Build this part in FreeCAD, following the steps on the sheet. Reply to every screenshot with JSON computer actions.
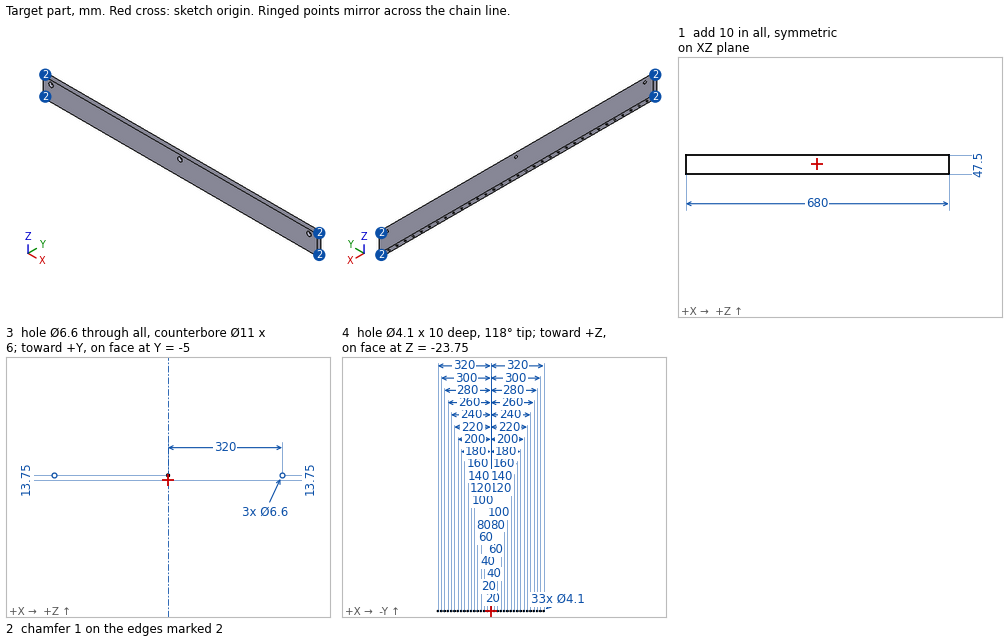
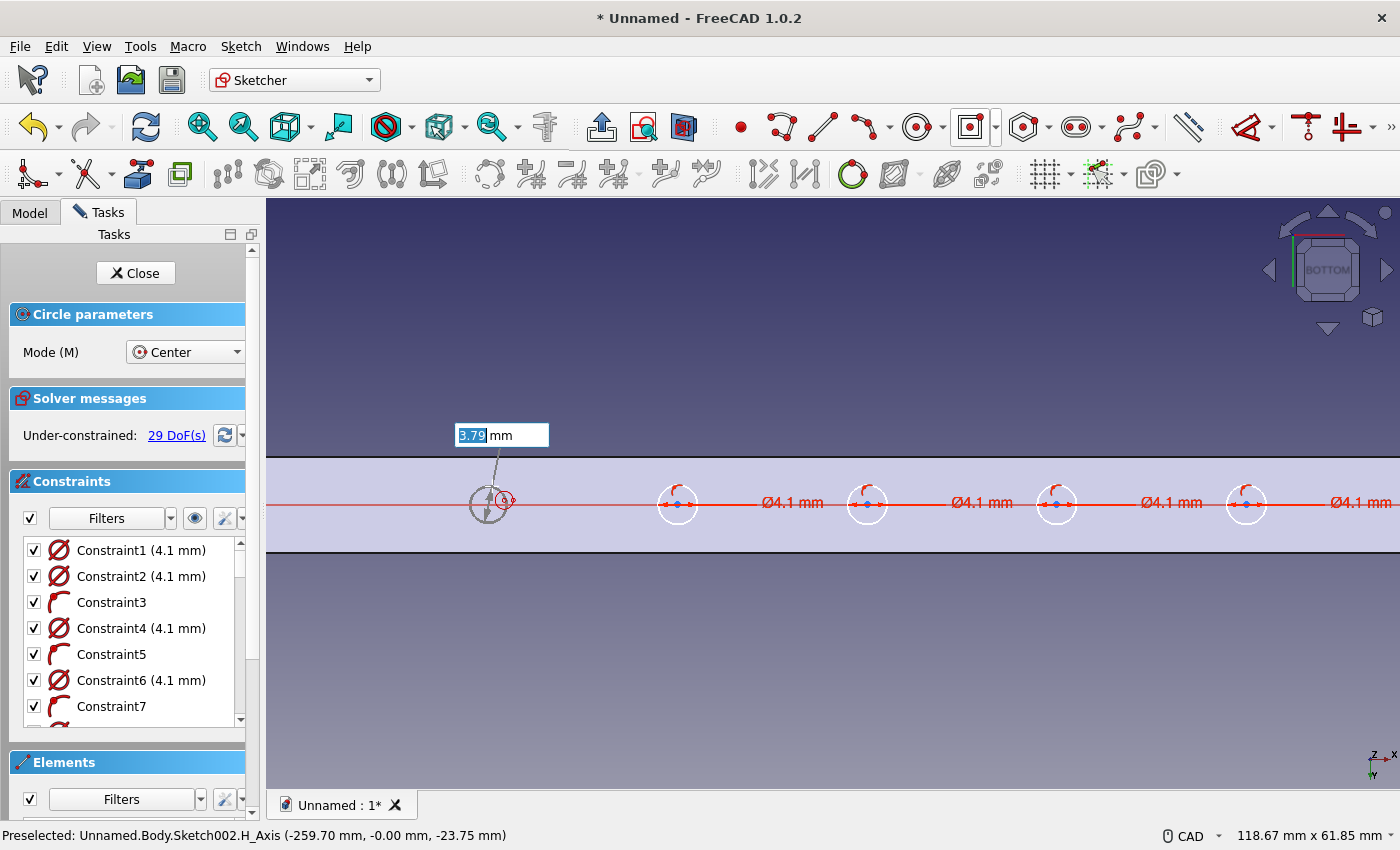
{"action": "type", "text": "4.1"}
{"action": "key", "text": "Return"}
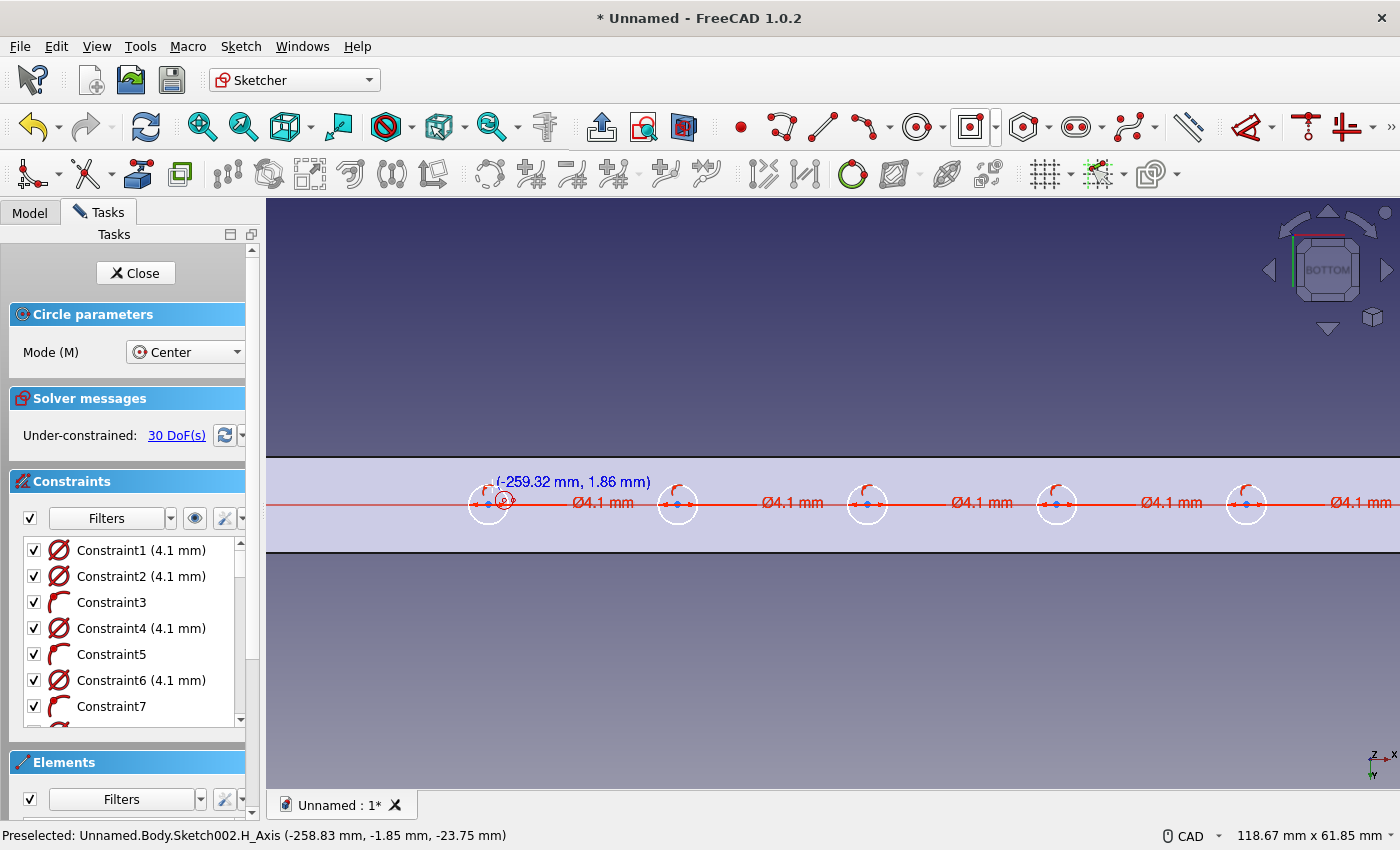
{"action": "scroll", "coordinate": [490, 492], "scroll_direction": "down", "scroll_amount": 11}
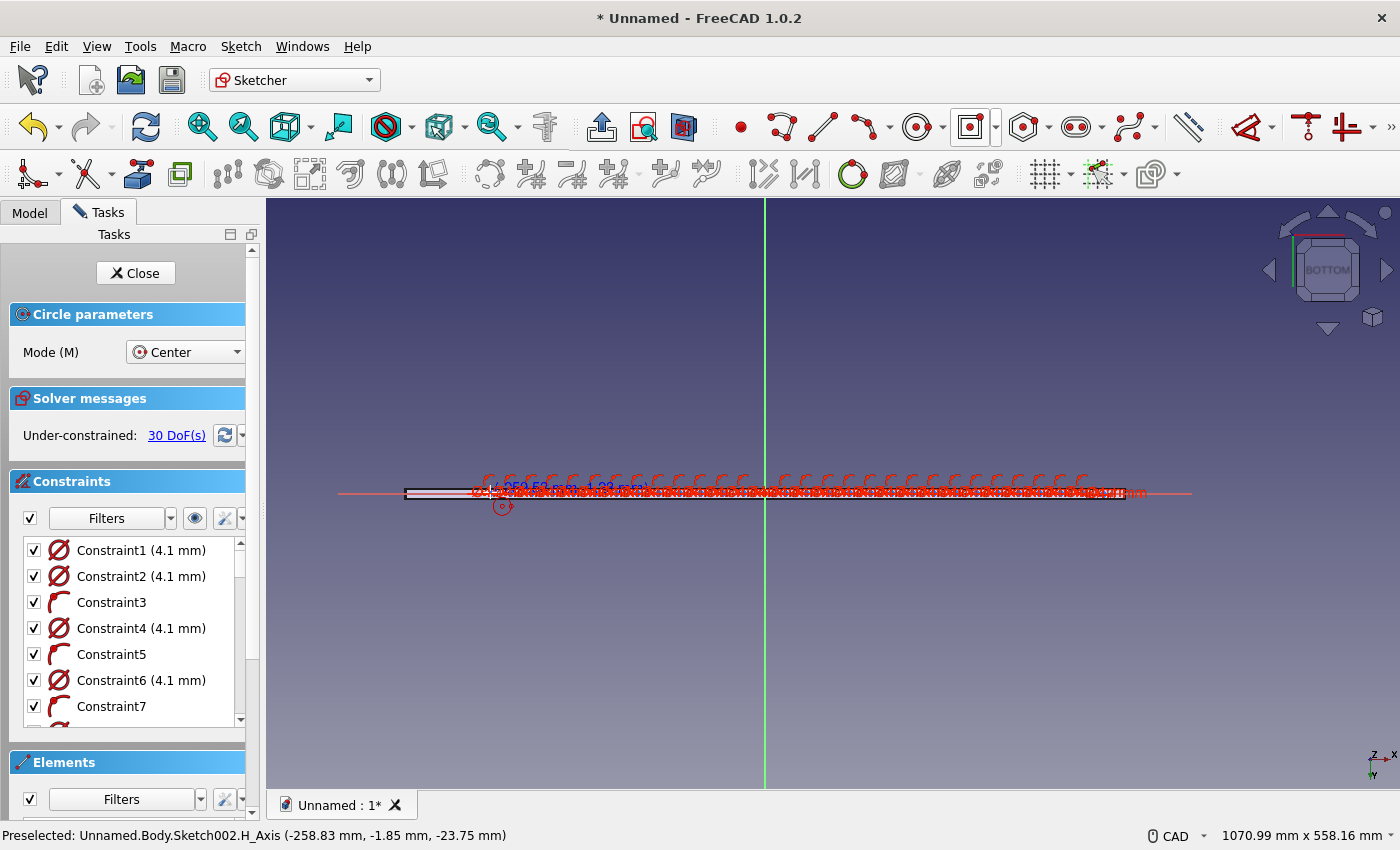
{"action": "left_click", "coordinate": [469, 494]}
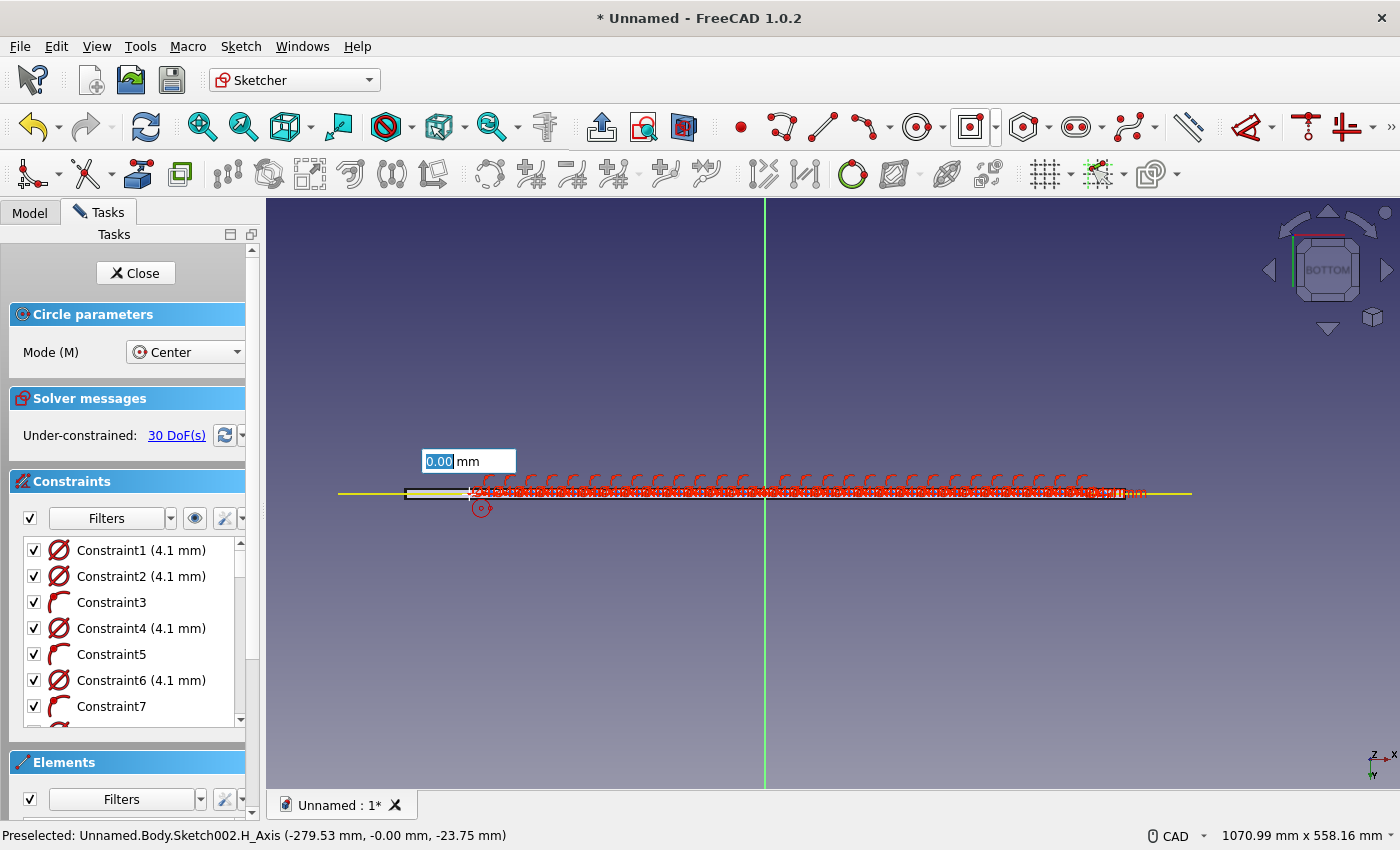
{"action": "scroll", "coordinate": [468, 496], "scroll_direction": "up", "scroll_amount": 11}
{"action": "mouse_move", "coordinate": [464, 491]}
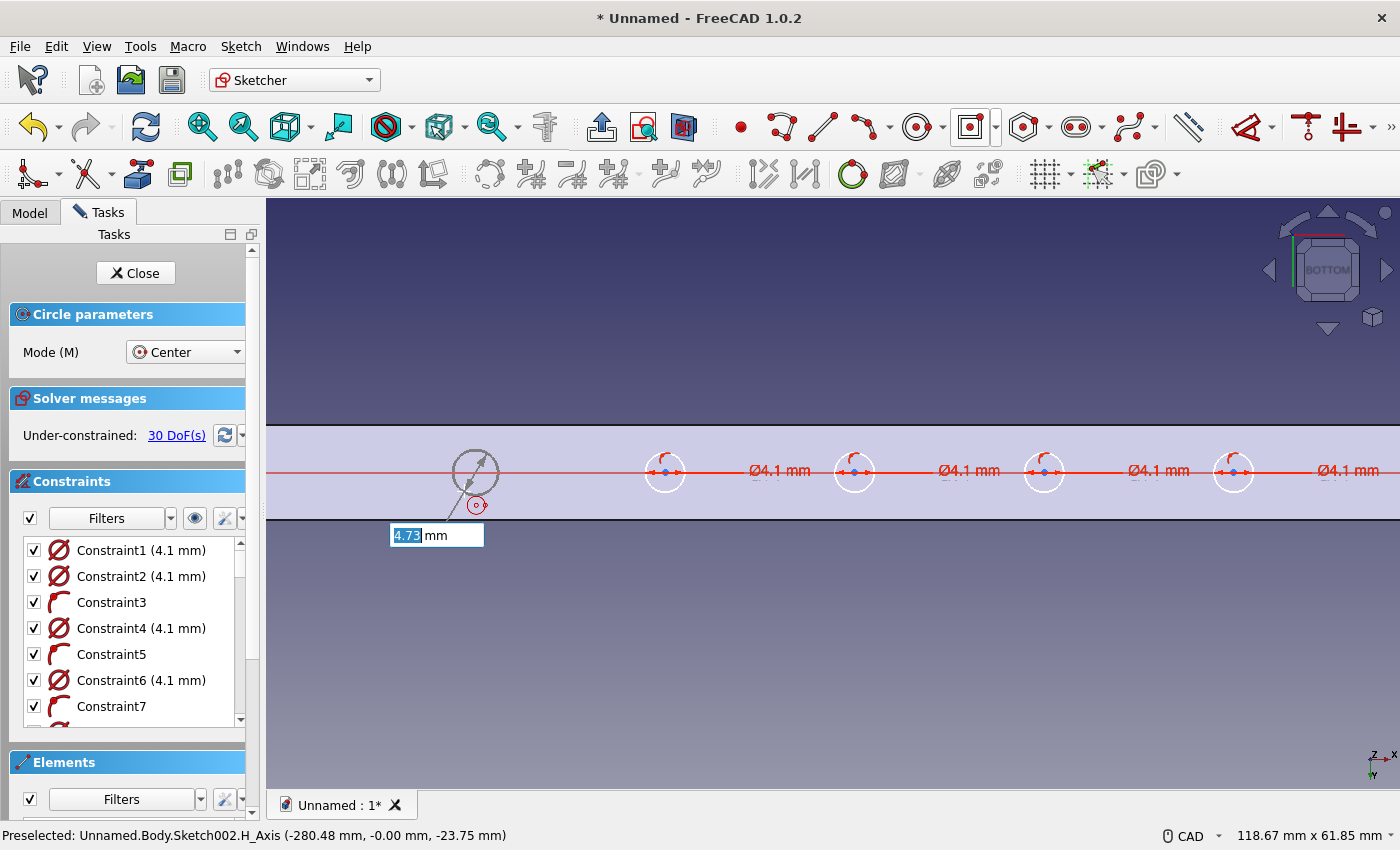
{"action": "type", "text": "4.1"}
{"action": "key", "text": "Return"}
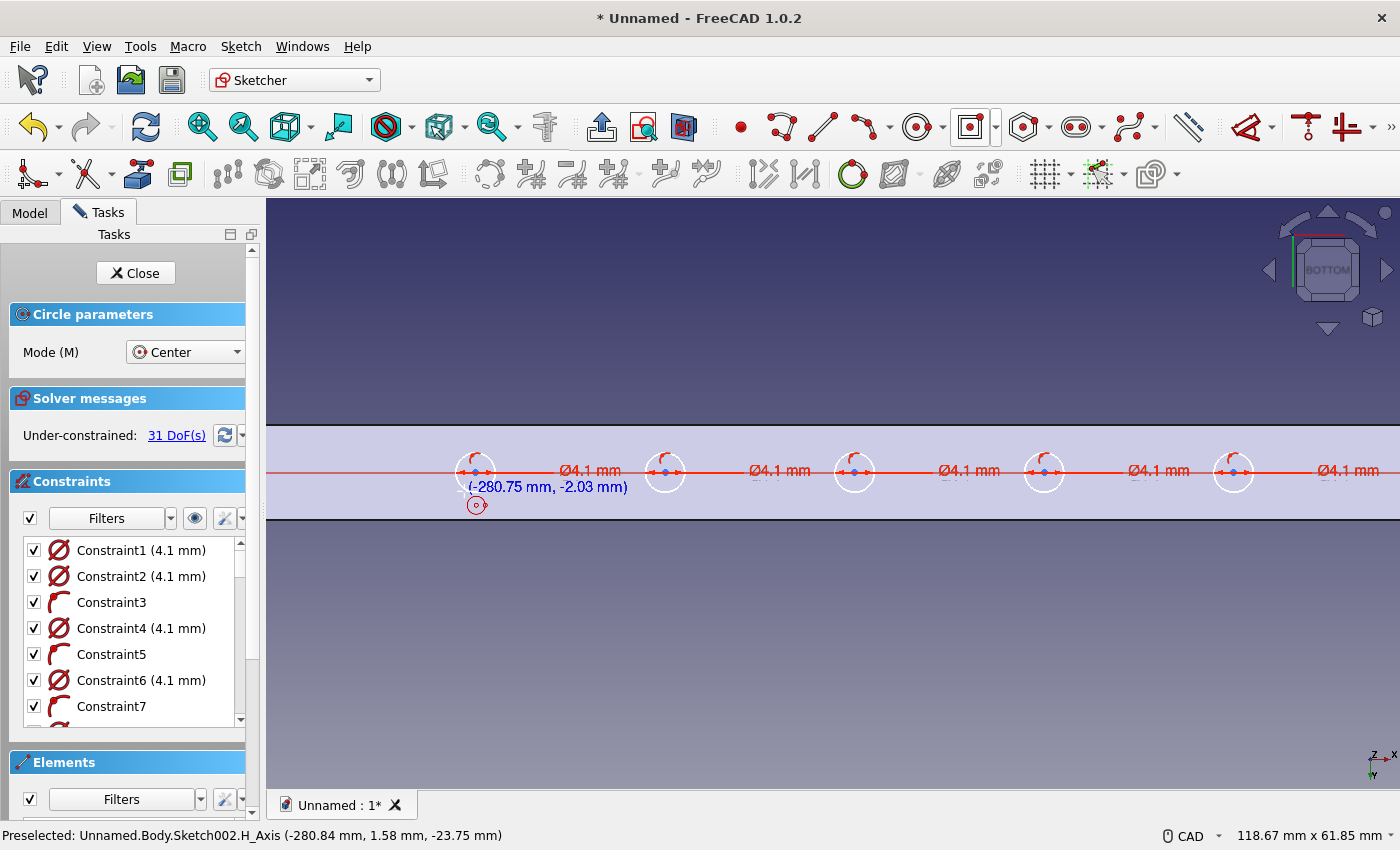
{"action": "scroll", "coordinate": [468, 496], "scroll_direction": "down", "scroll_amount": 11}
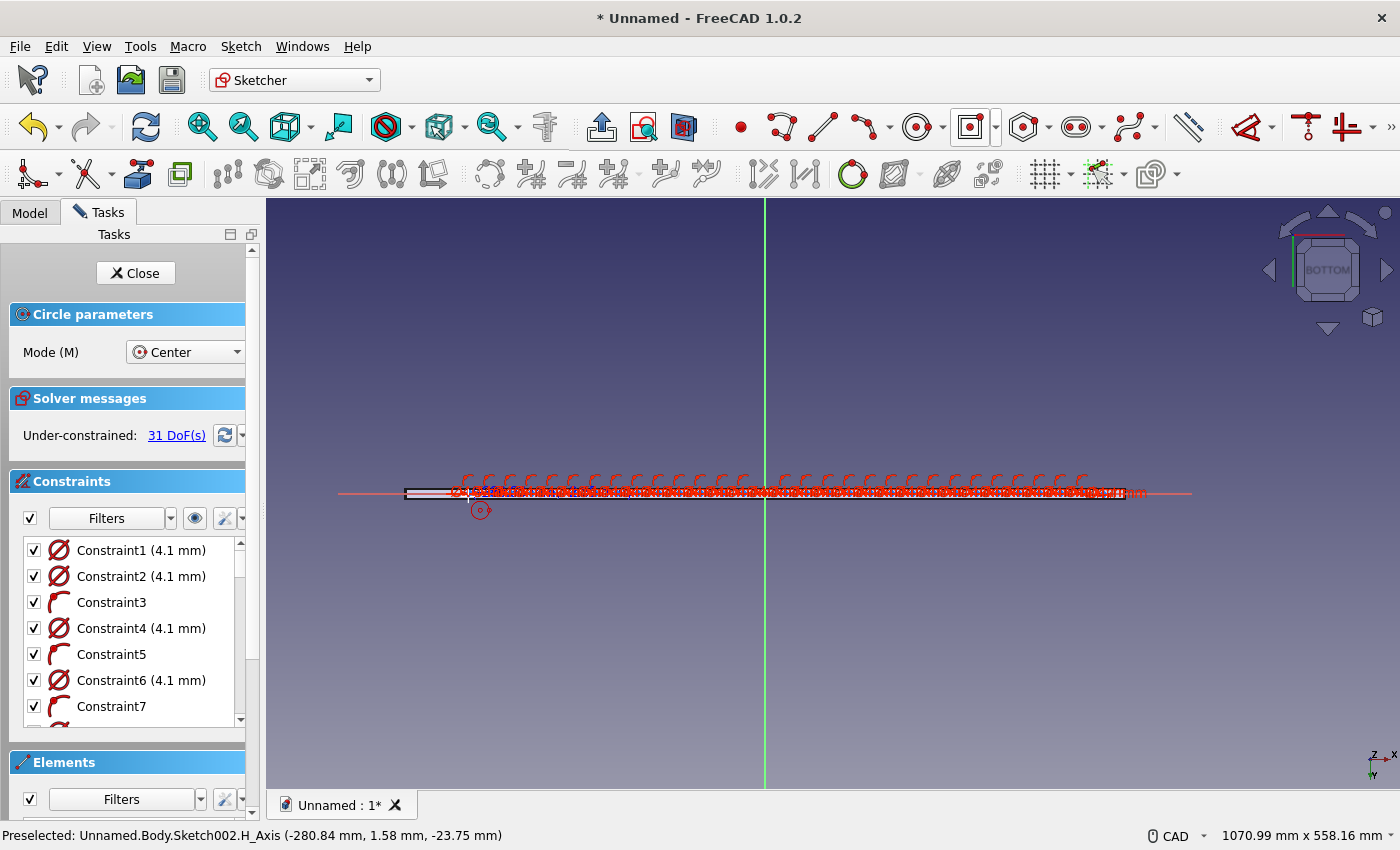
{"action": "scroll", "coordinate": [447, 494], "scroll_direction": "up", "scroll_amount": 12}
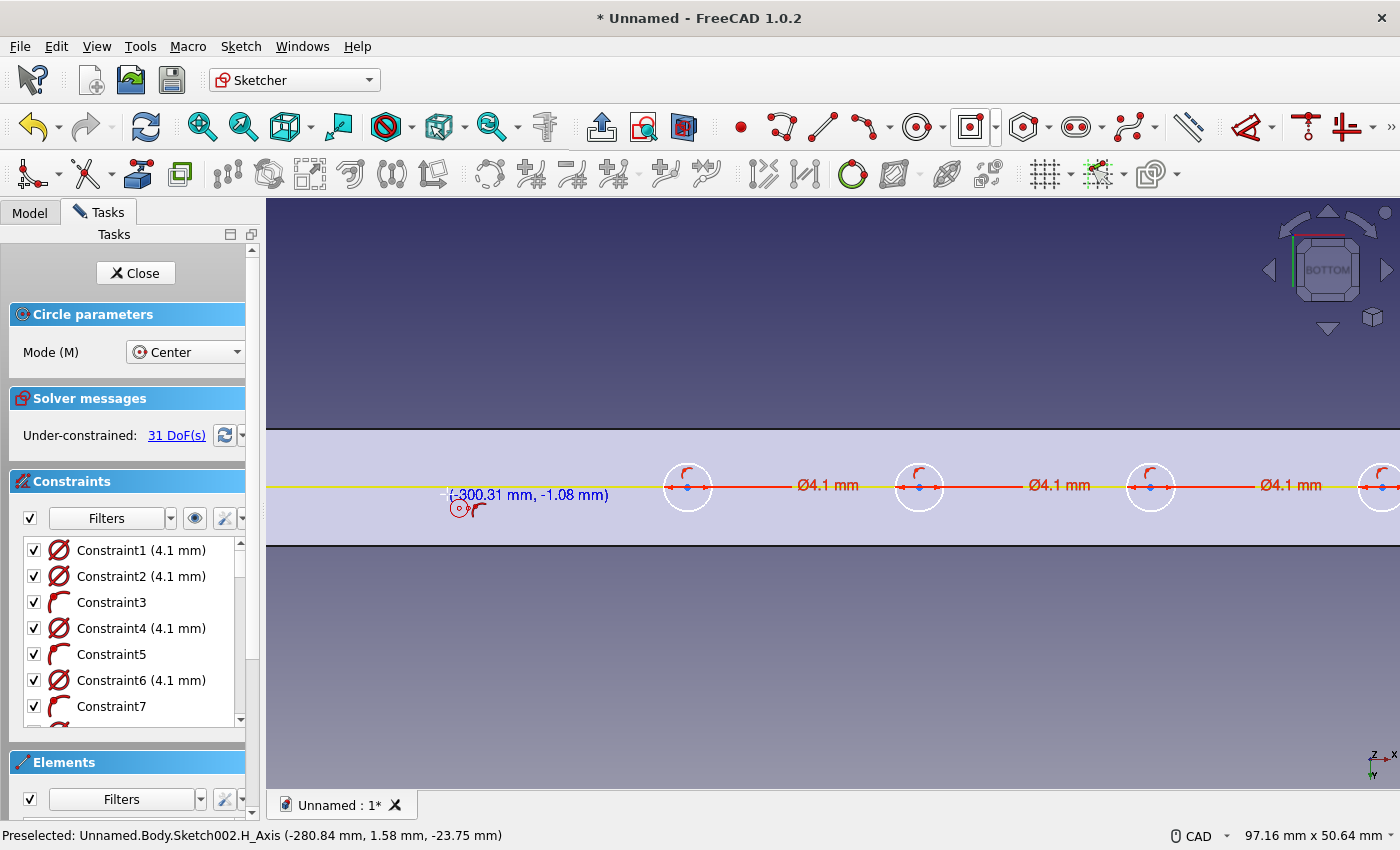
{"action": "scroll", "coordinate": [447, 494], "scroll_direction": "down", "scroll_amount": 12}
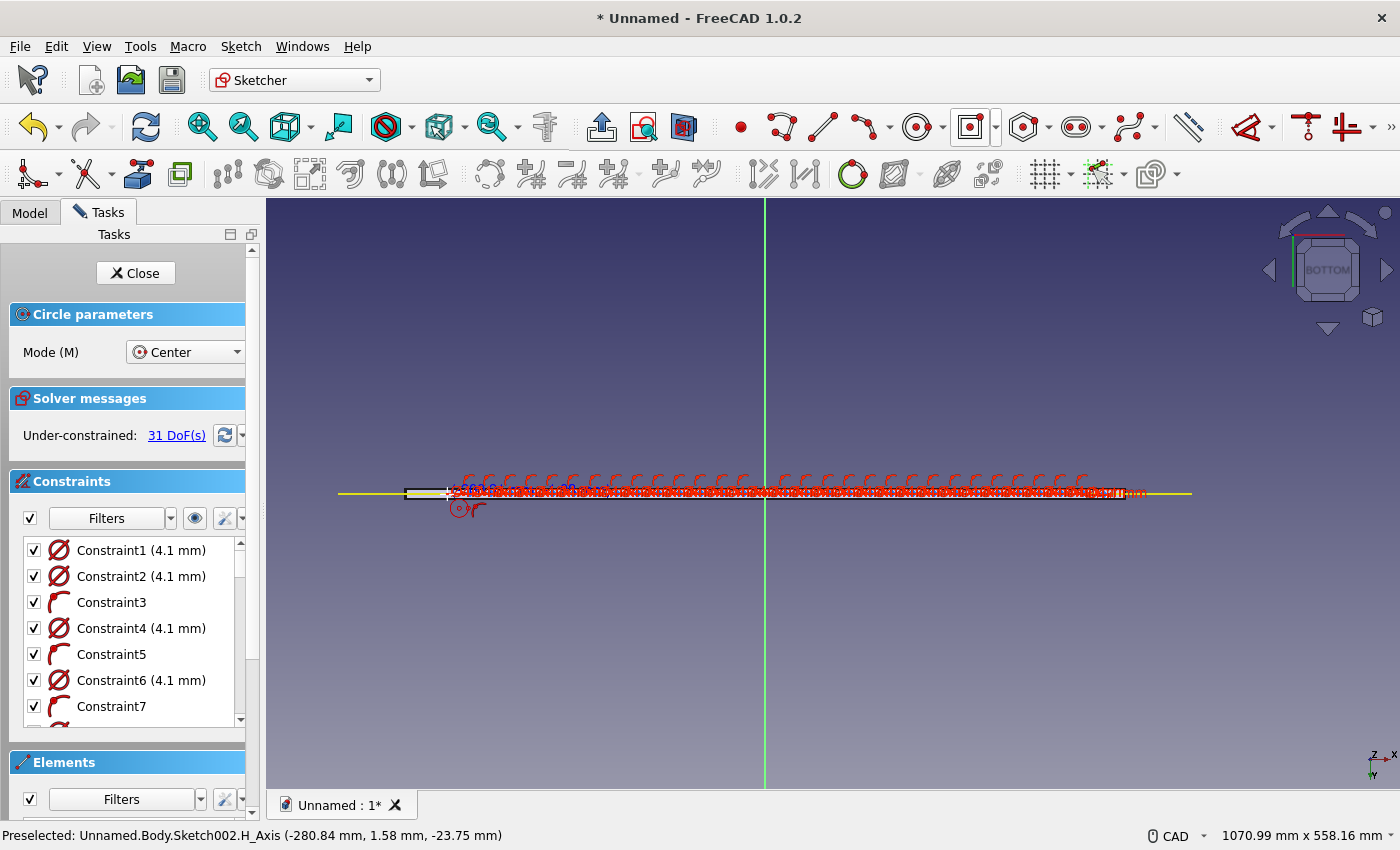
{"action": "left_click", "coordinate": [447, 494]}